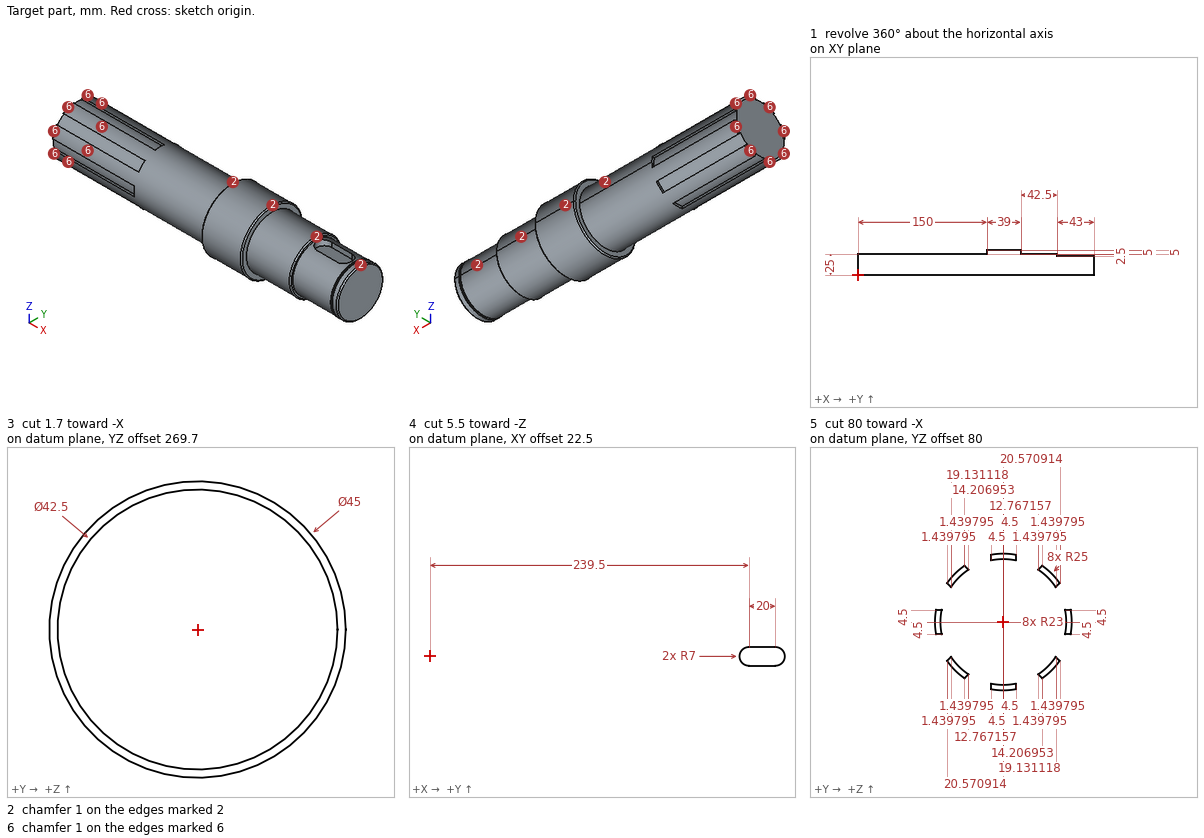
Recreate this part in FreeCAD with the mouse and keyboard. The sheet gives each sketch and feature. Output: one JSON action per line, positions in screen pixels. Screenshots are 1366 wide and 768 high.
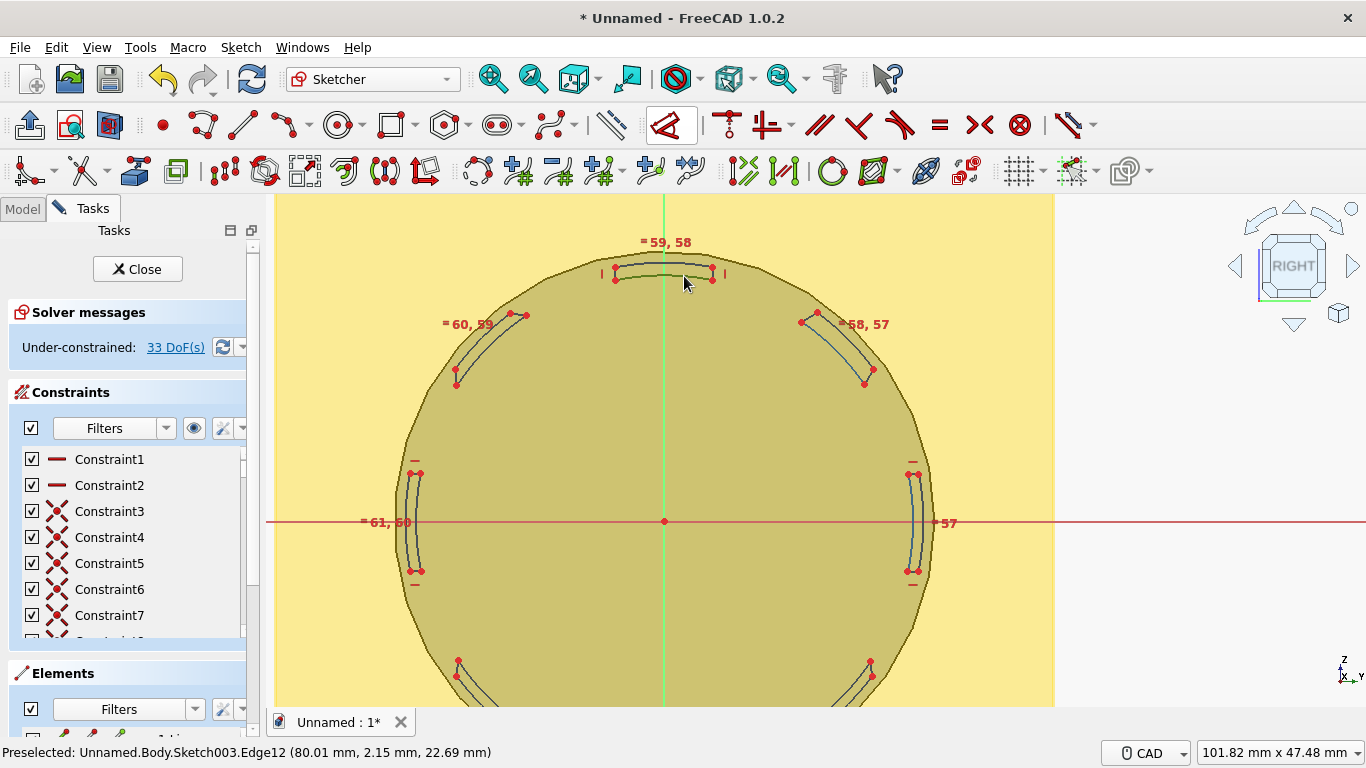
{"action": "scroll", "coordinate": [503, 334], "scroll_direction": "up", "scroll_amount": 2}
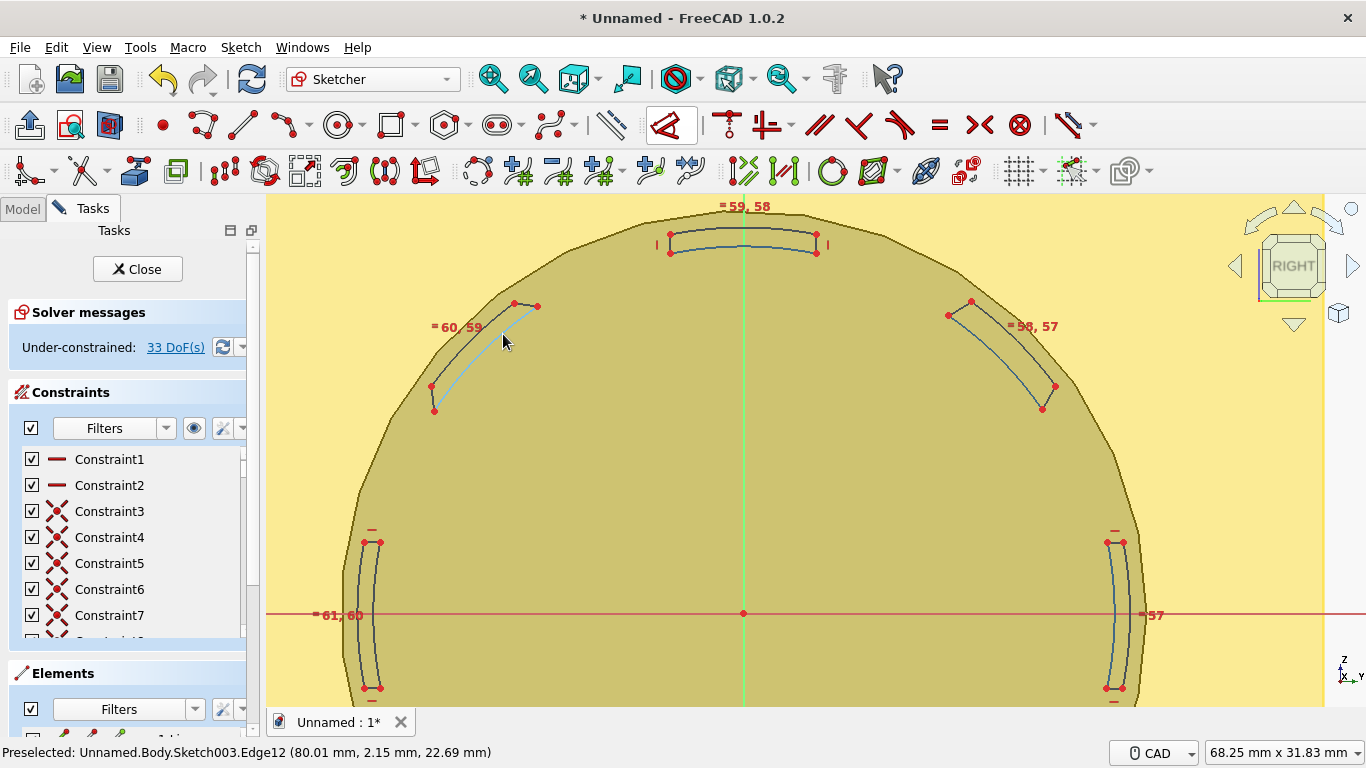
{"action": "left_click", "coordinate": [502, 333]}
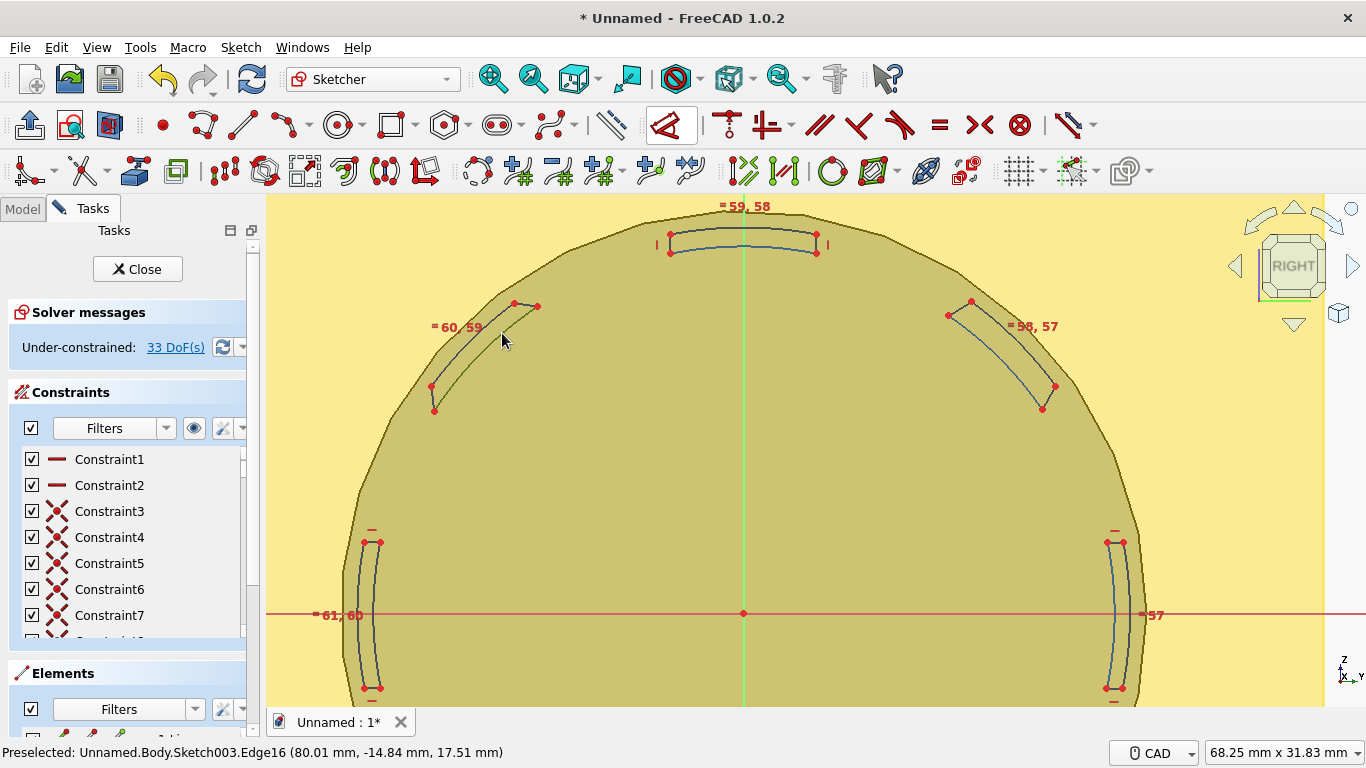
{"action": "left_click", "coordinate": [374, 586]}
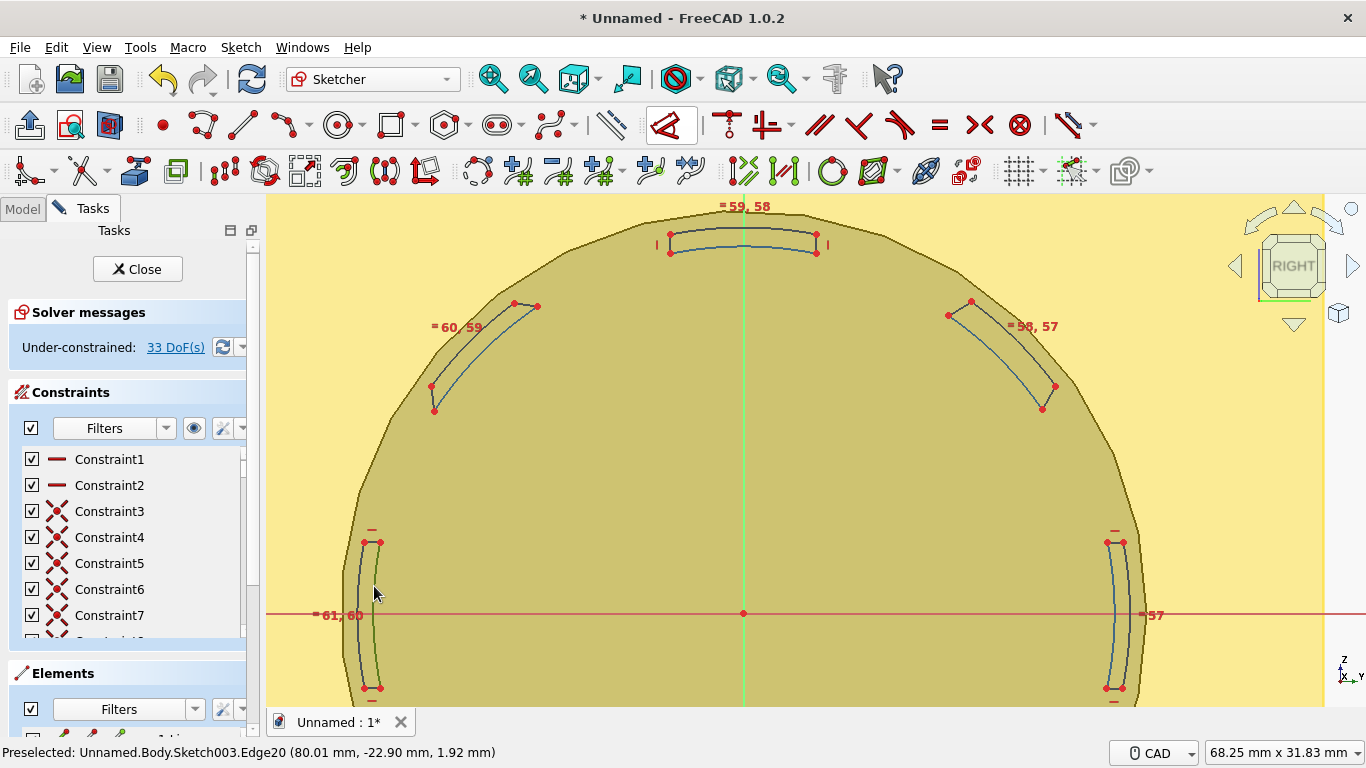
{"action": "scroll", "coordinate": [750, 355], "scroll_direction": "down", "scroll_amount": 5}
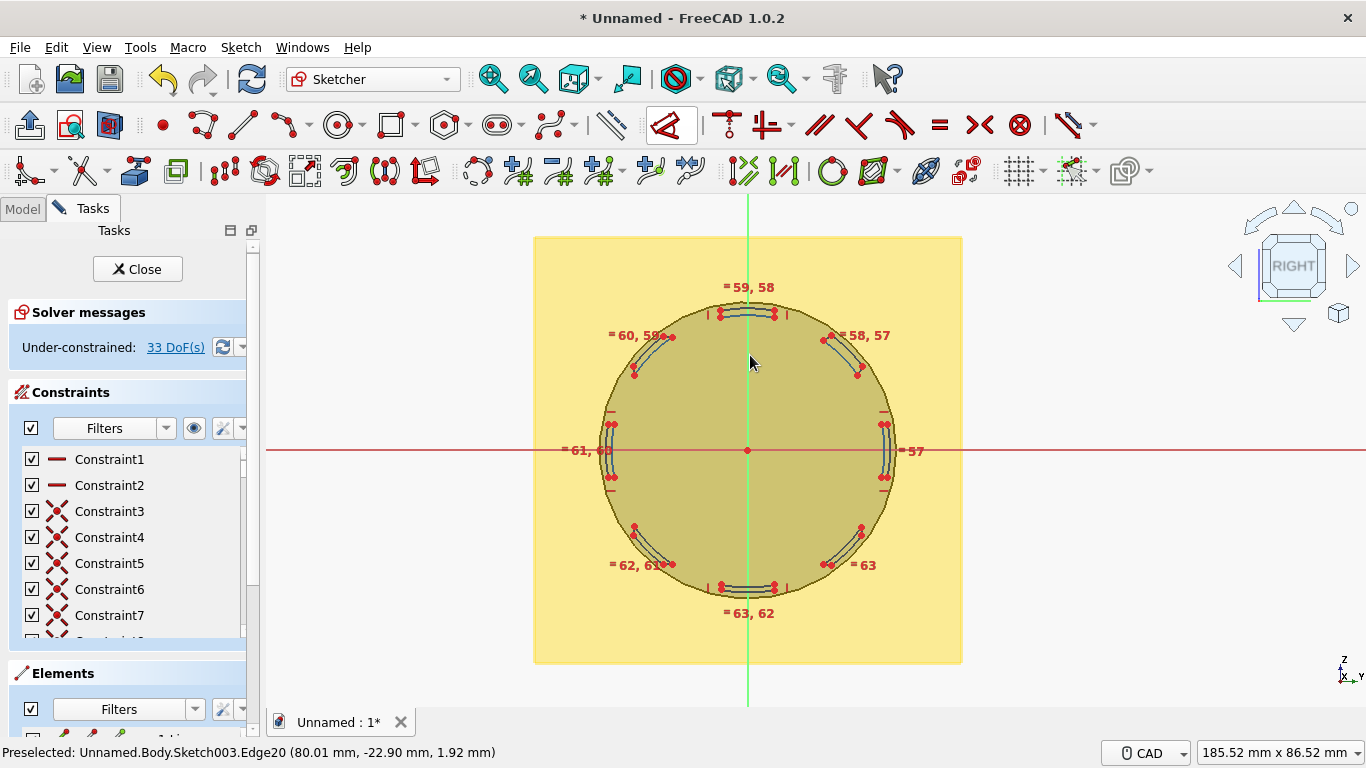
{"action": "scroll", "coordinate": [644, 539], "scroll_direction": "up", "scroll_amount": 5}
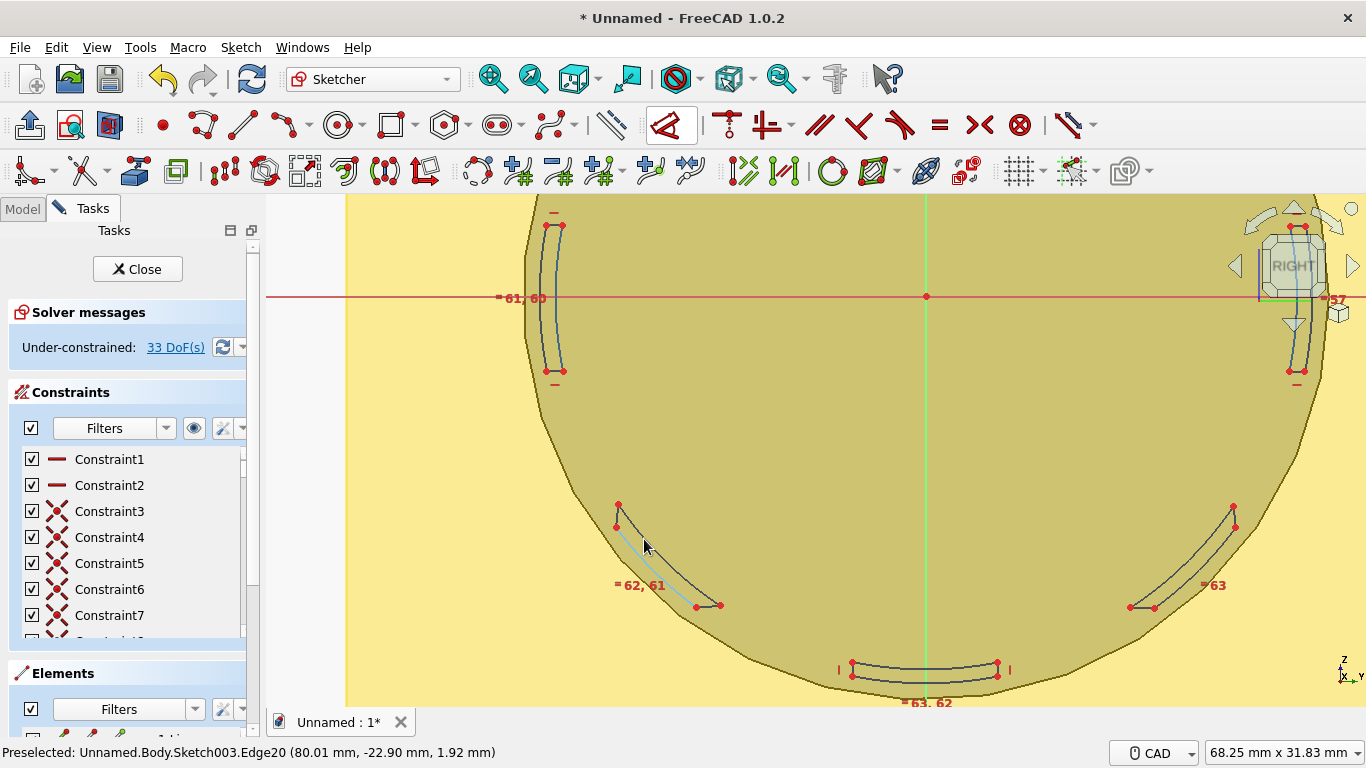
{"action": "left_click", "coordinate": [645, 539]}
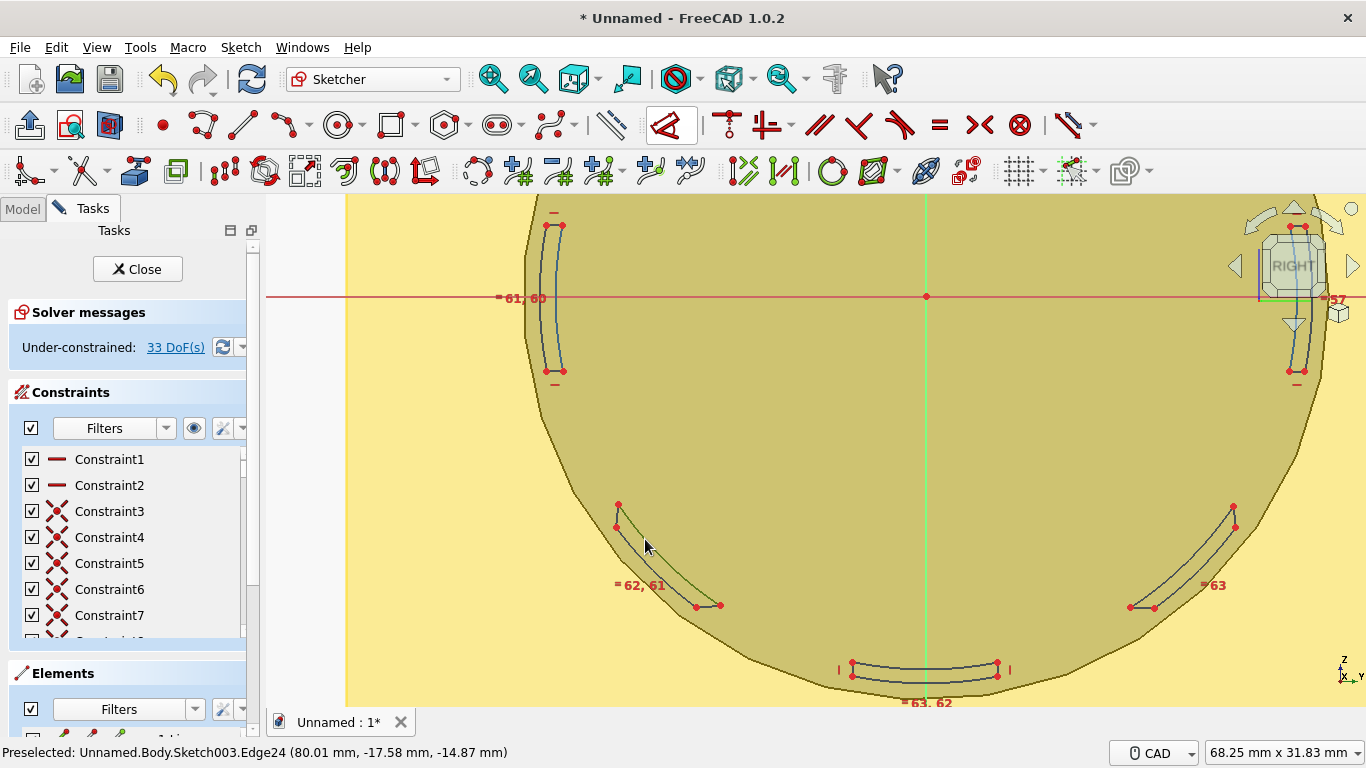
{"action": "left_click", "coordinate": [896, 668]}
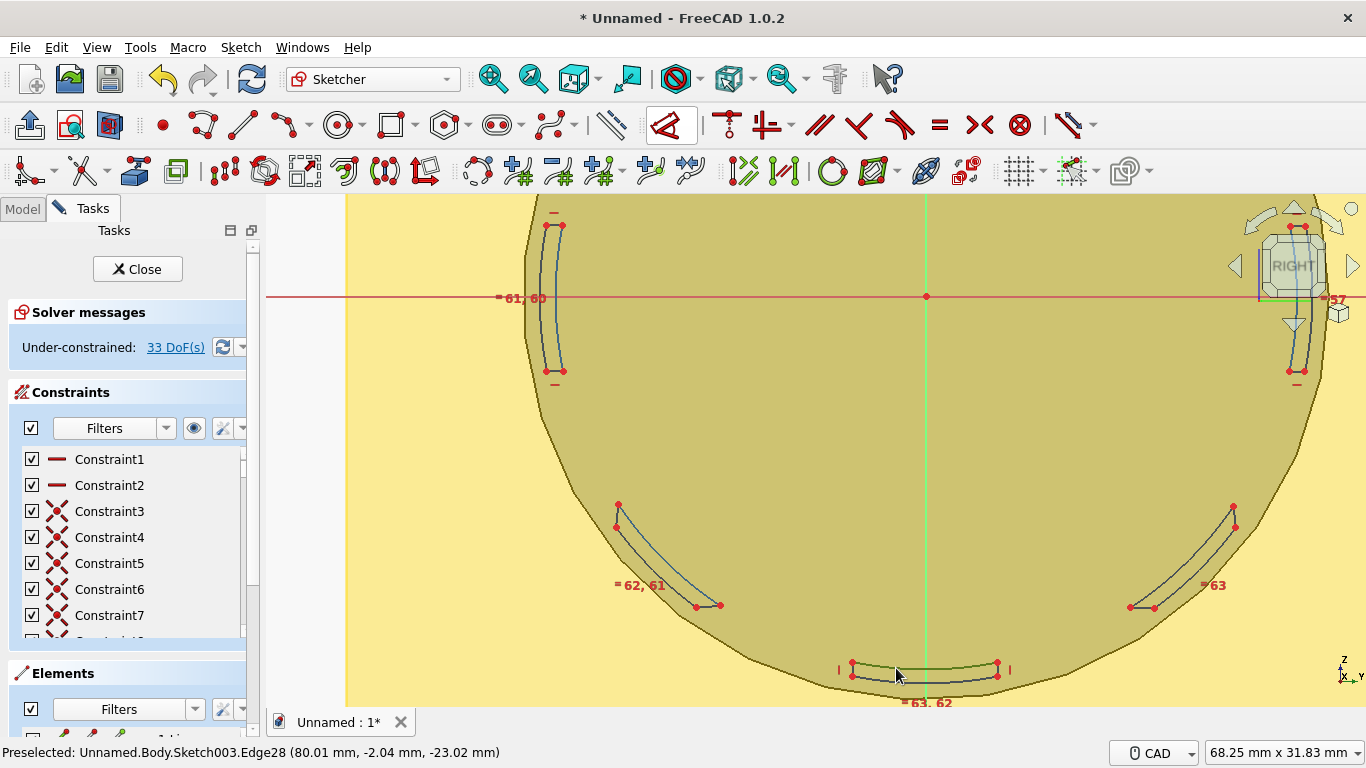
{"action": "left_click", "coordinate": [1166, 581]}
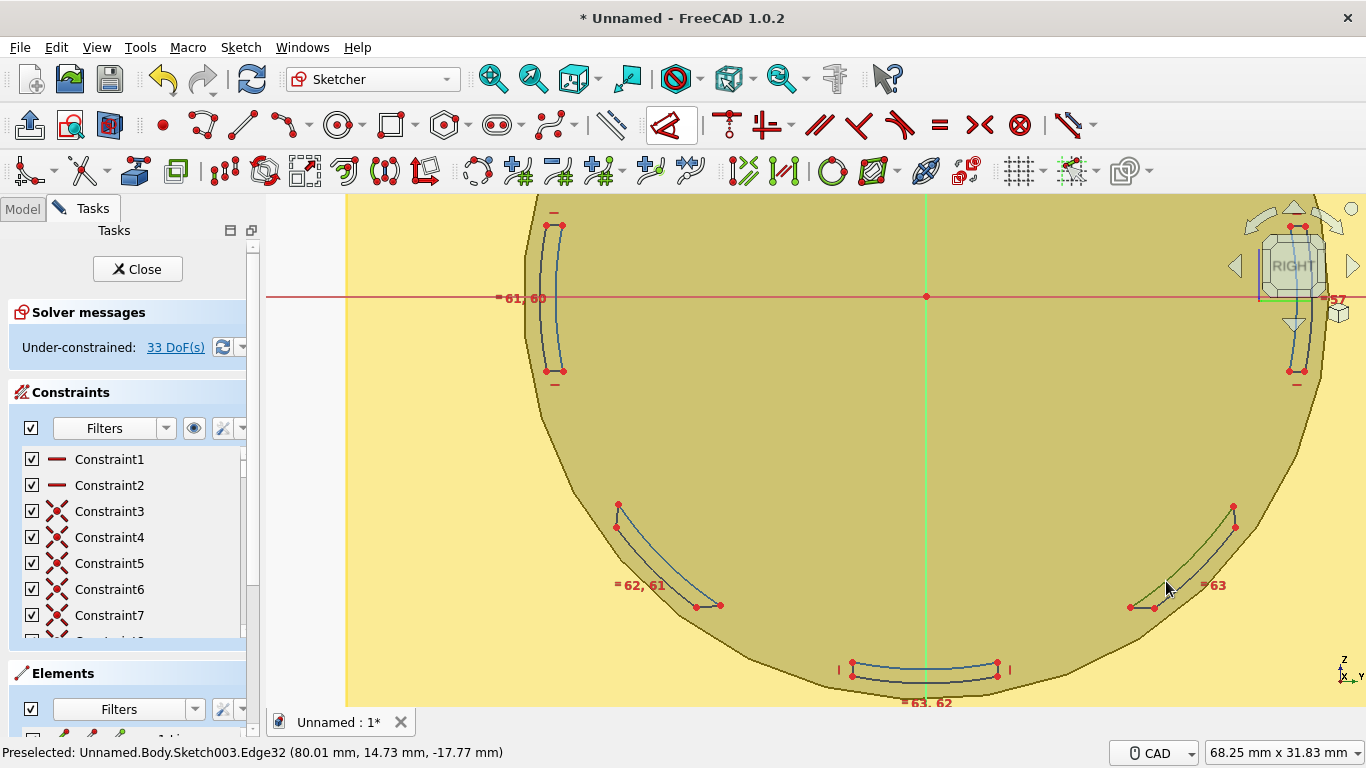
{"action": "key", "text": "e"}